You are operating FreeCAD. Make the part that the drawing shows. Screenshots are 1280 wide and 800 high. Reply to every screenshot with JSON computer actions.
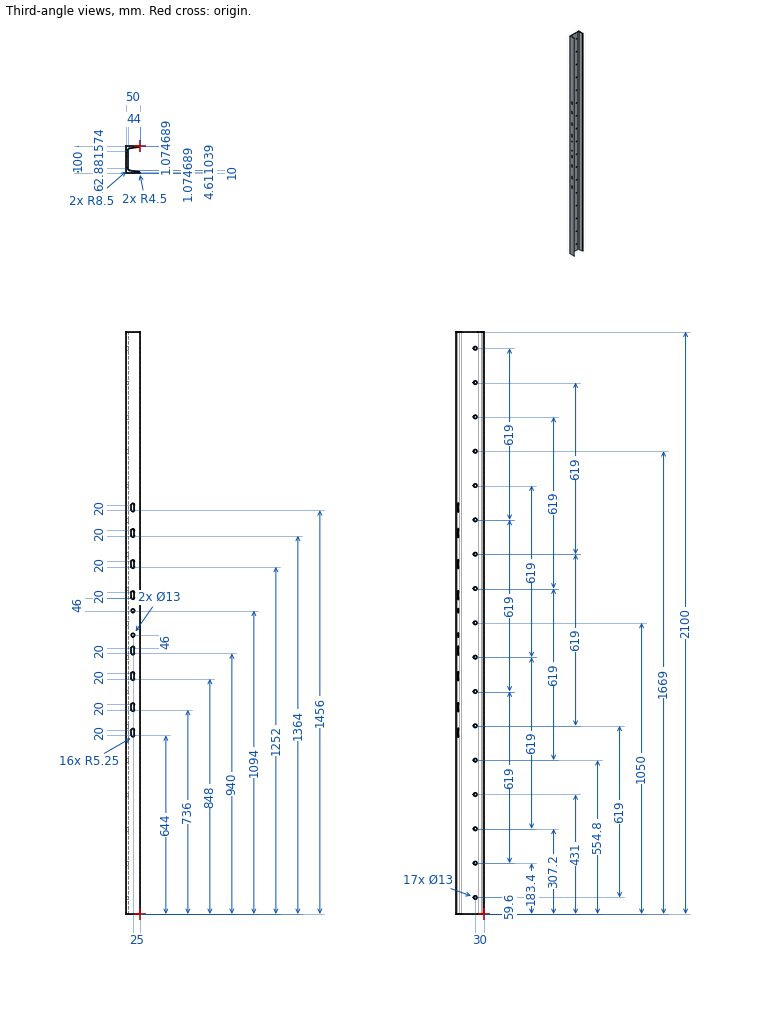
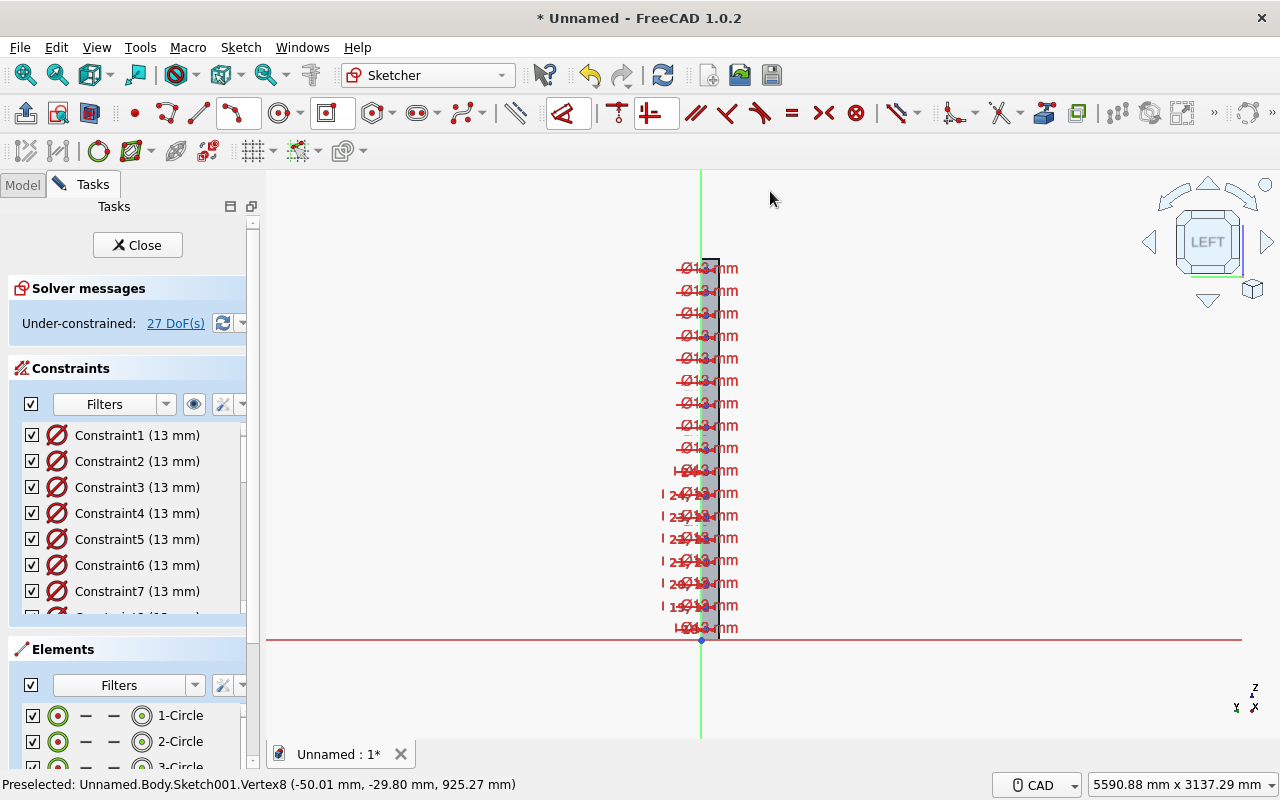
{"action": "left_click", "coordinate": [707, 472]}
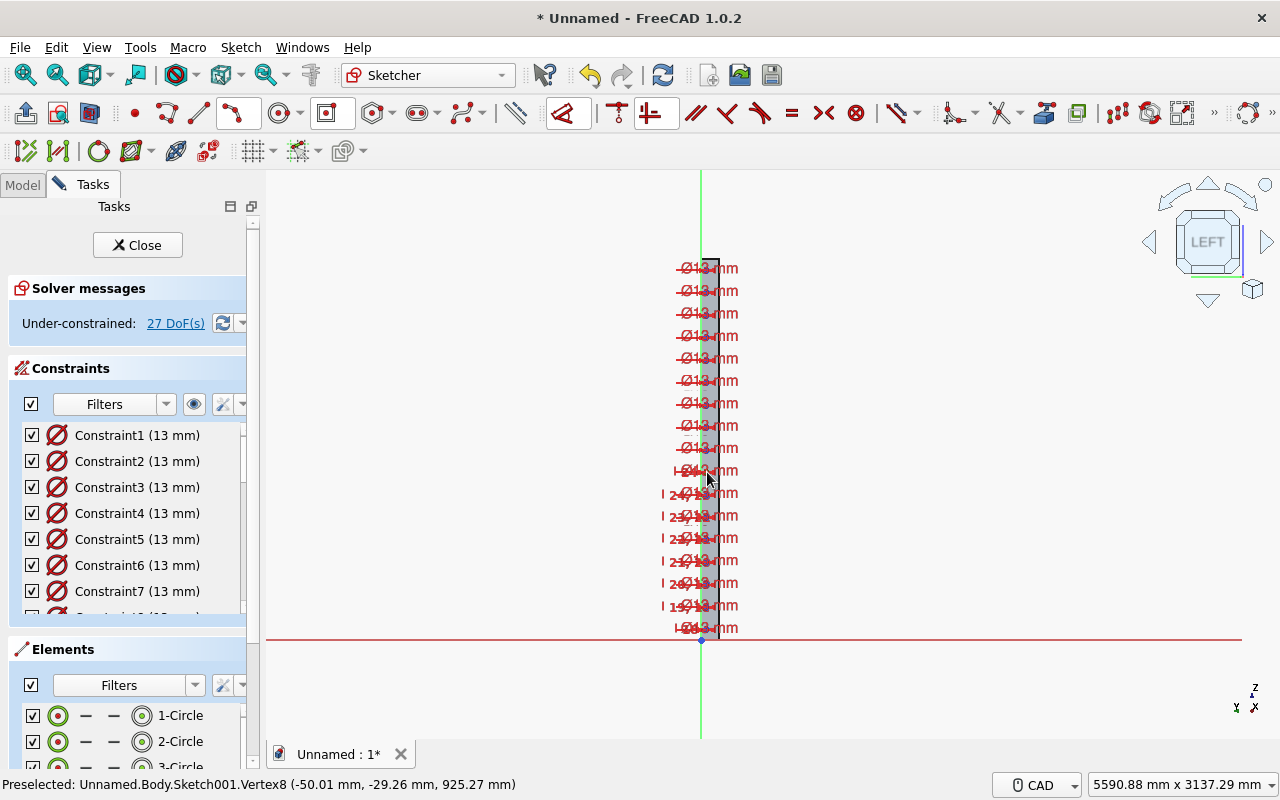
{"action": "left_click", "coordinate": [707, 450]}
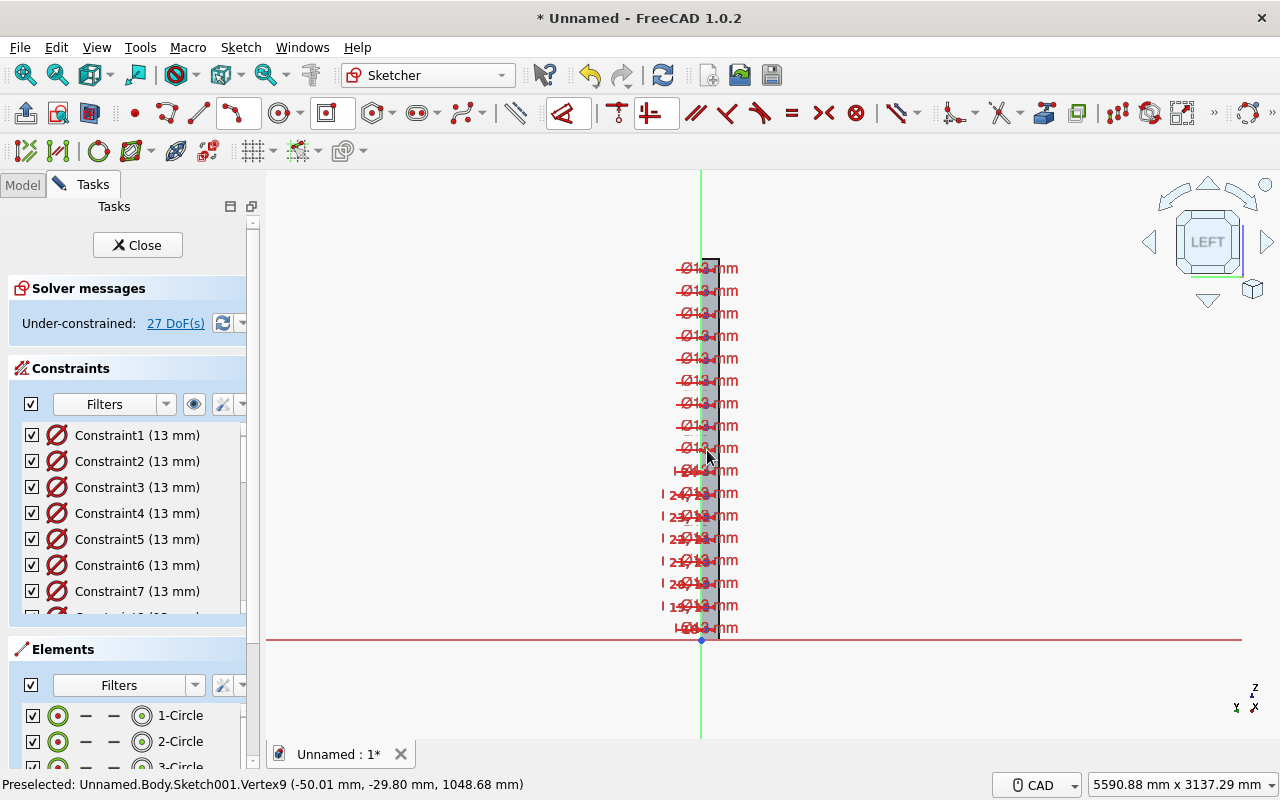
{"action": "key", "text": "v"}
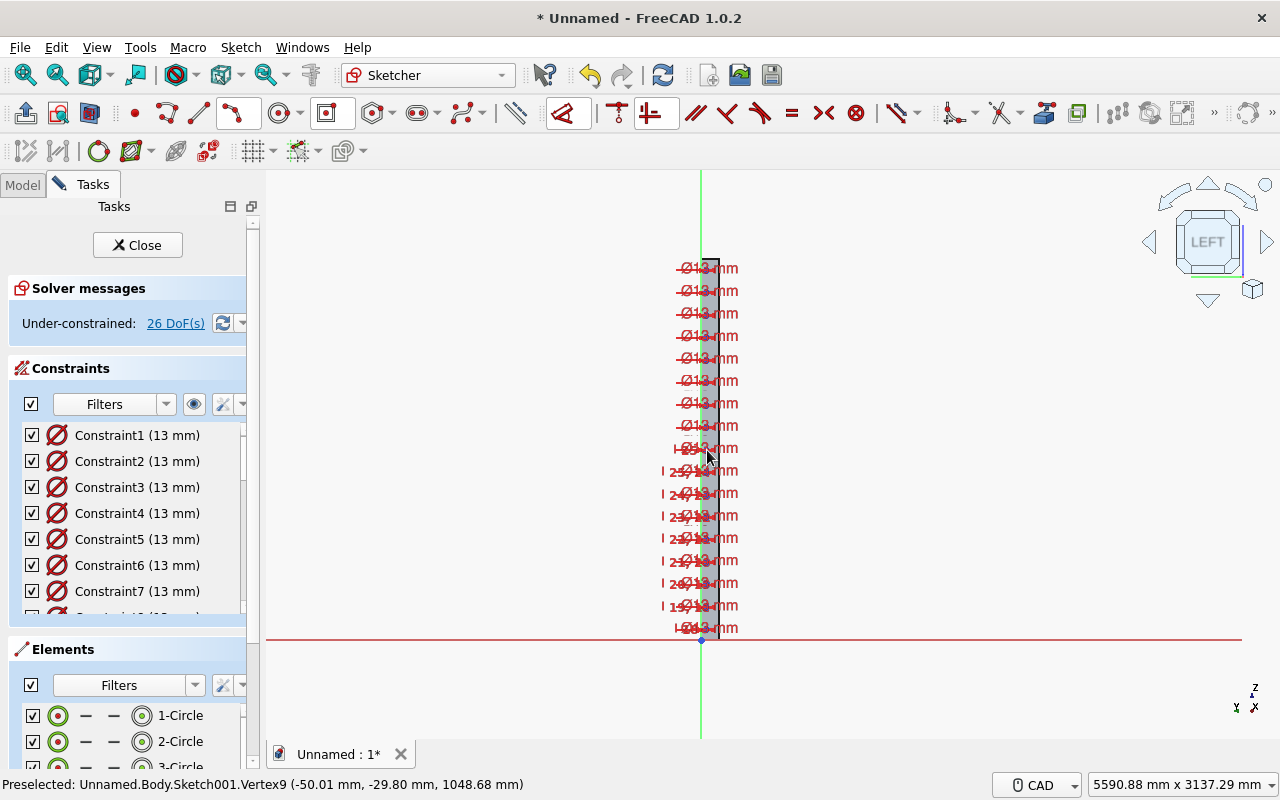
{"action": "left_click", "coordinate": [707, 450]}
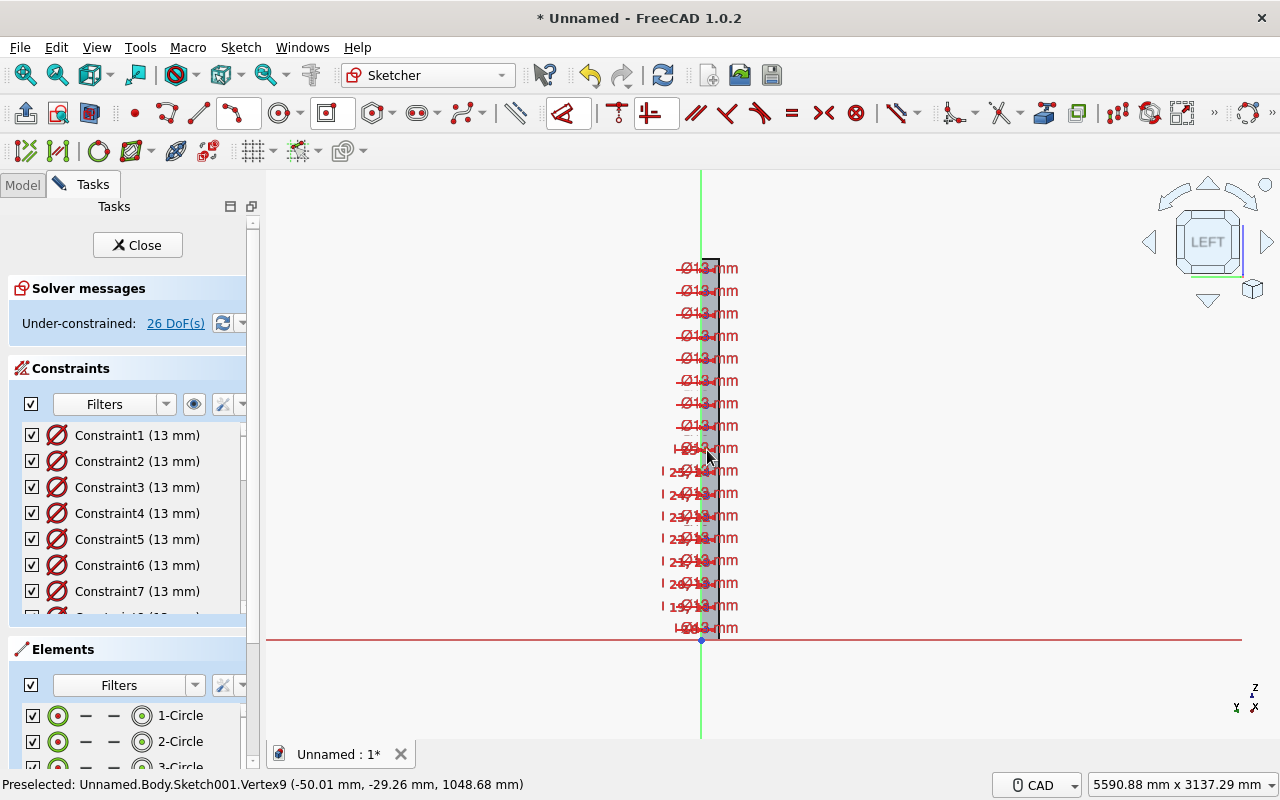
{"action": "left_click", "coordinate": [707, 428]}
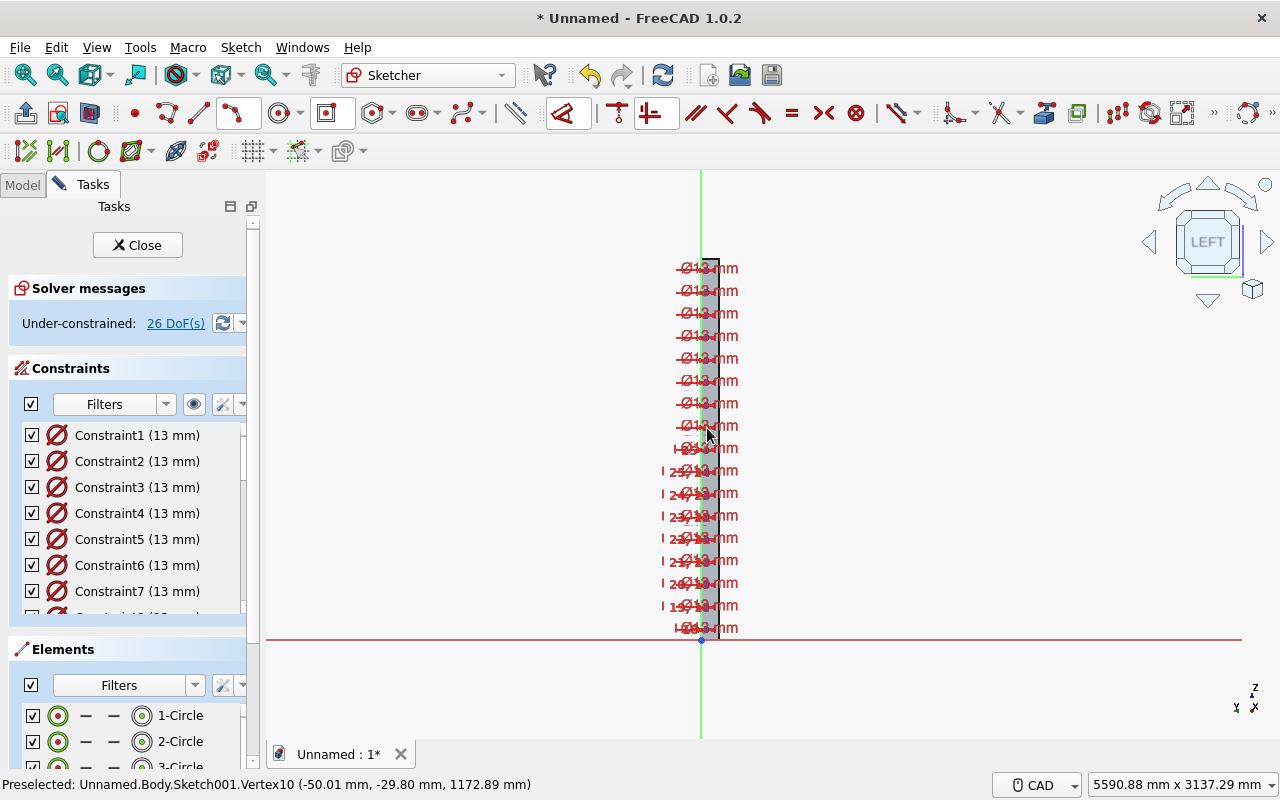
{"action": "key", "text": "v"}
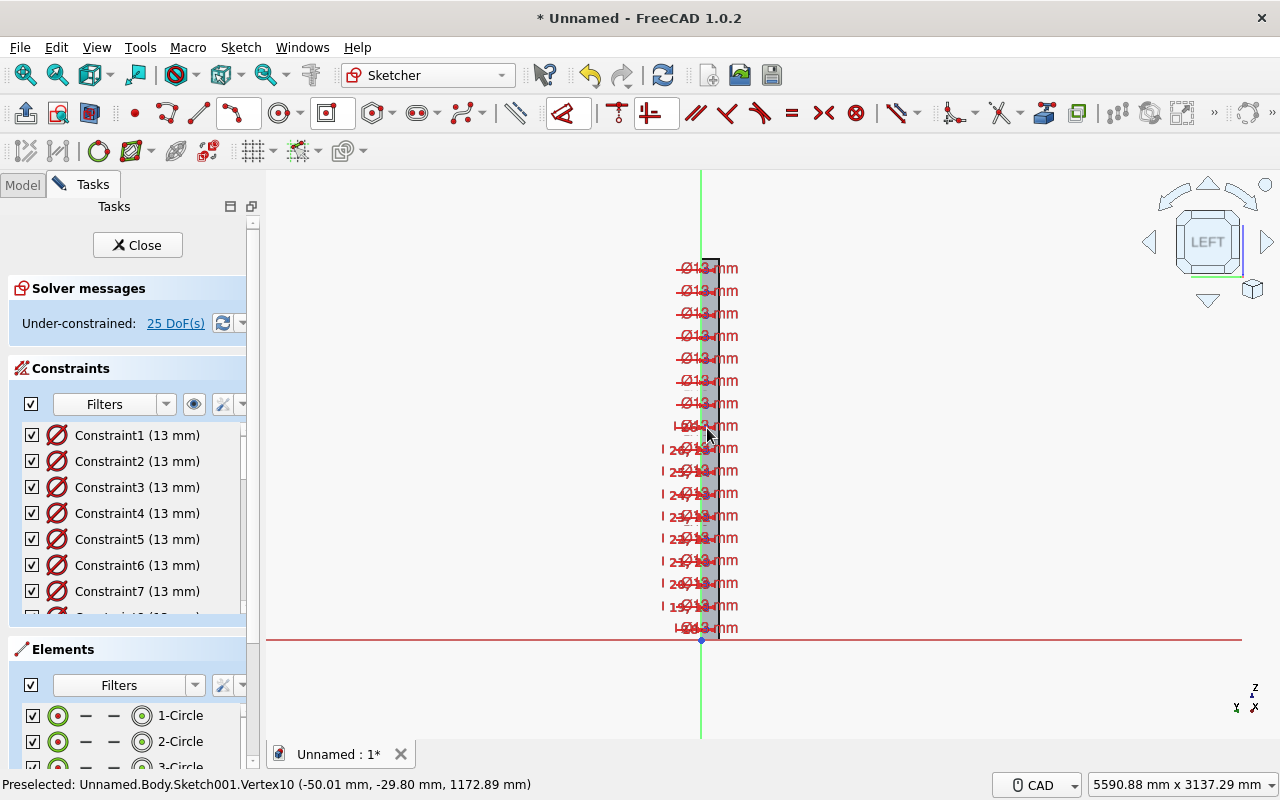
{"action": "left_click", "coordinate": [707, 428]}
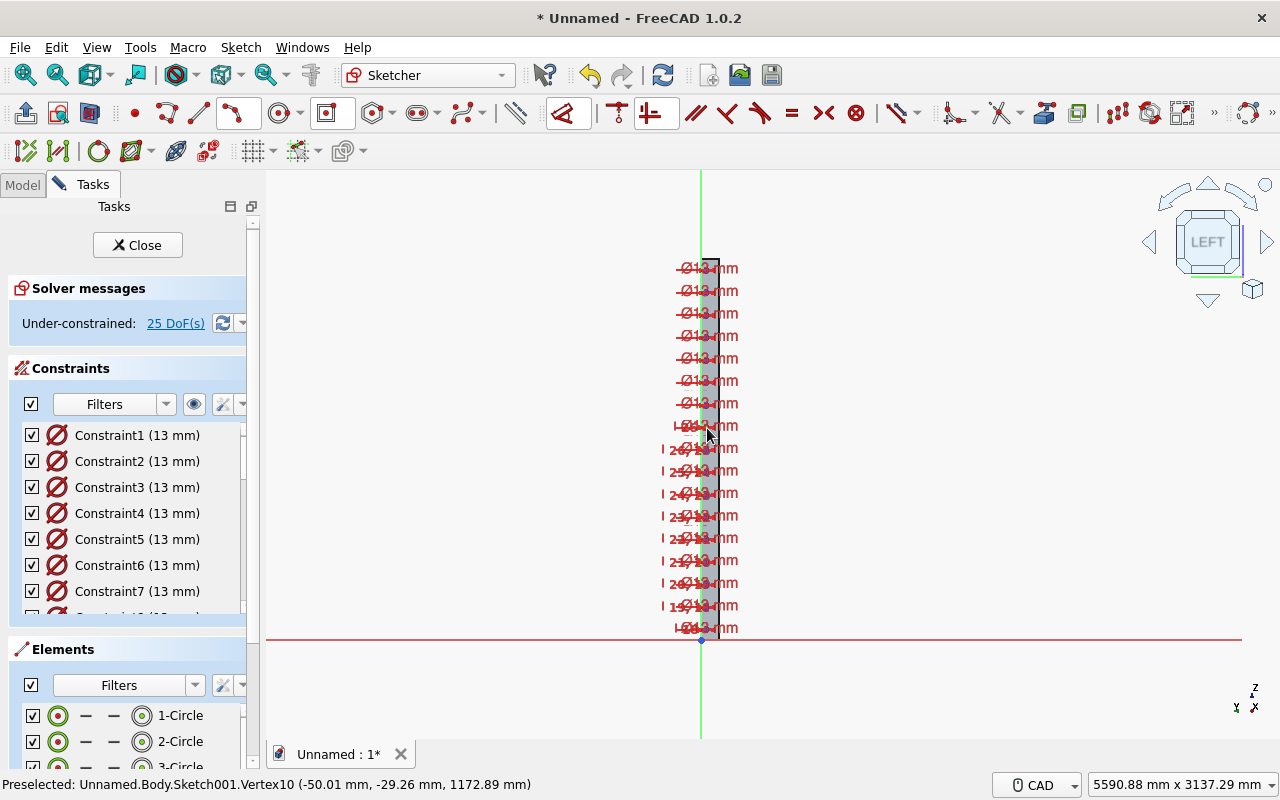
{"action": "left_click", "coordinate": [707, 405]}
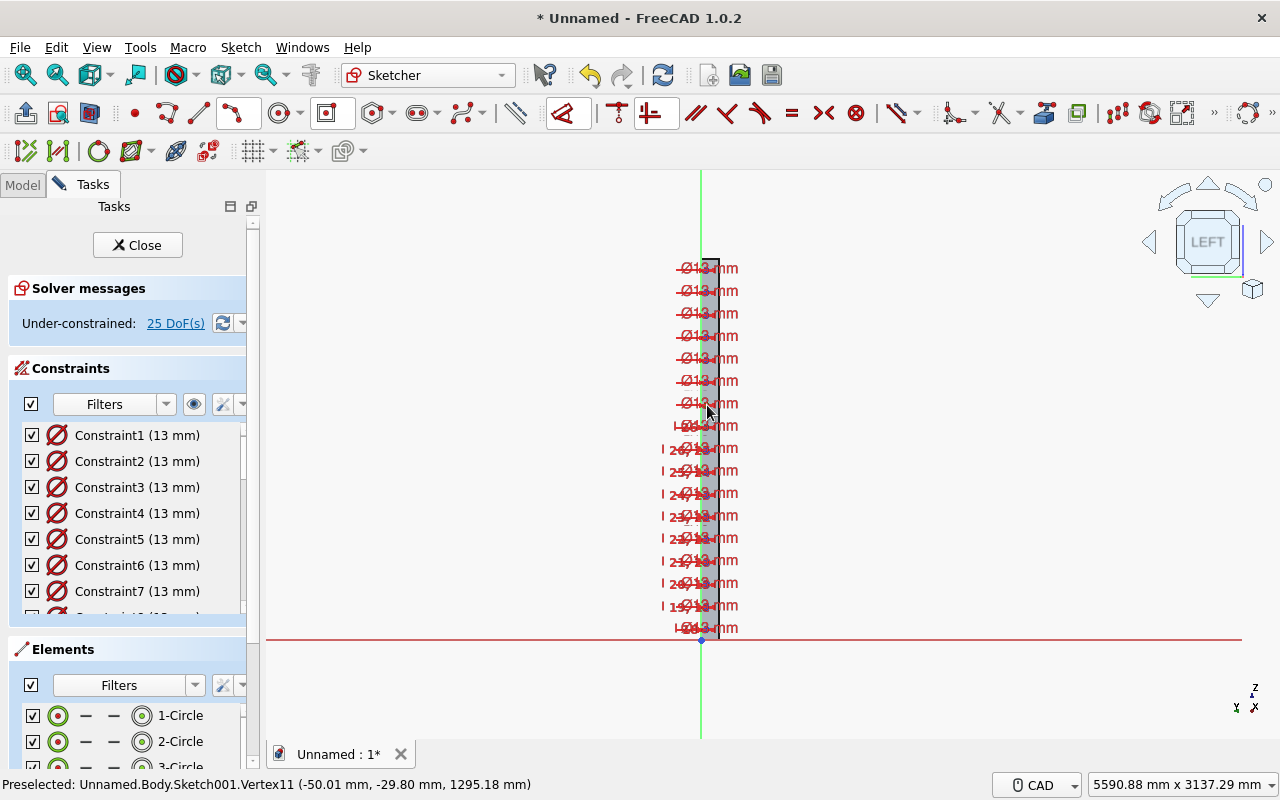
{"action": "key", "text": "v"}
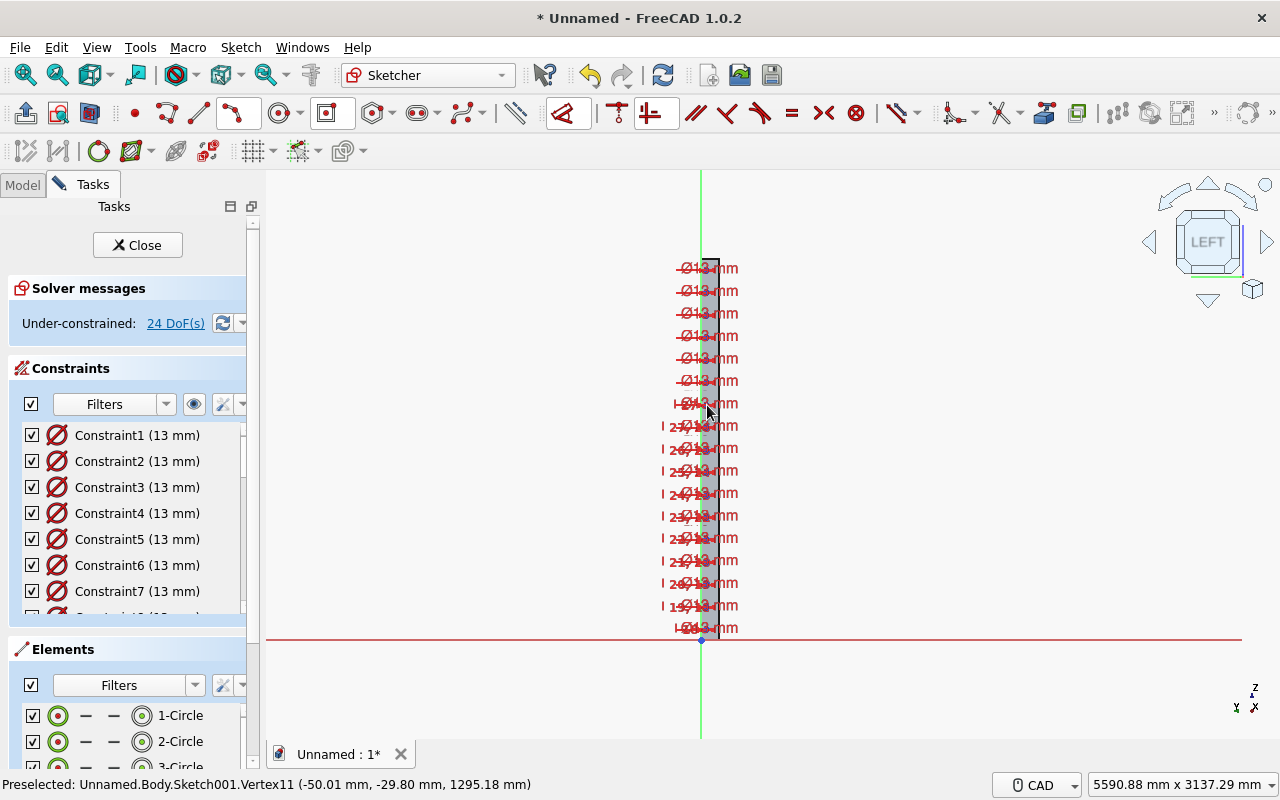
{"action": "left_click", "coordinate": [707, 405]}